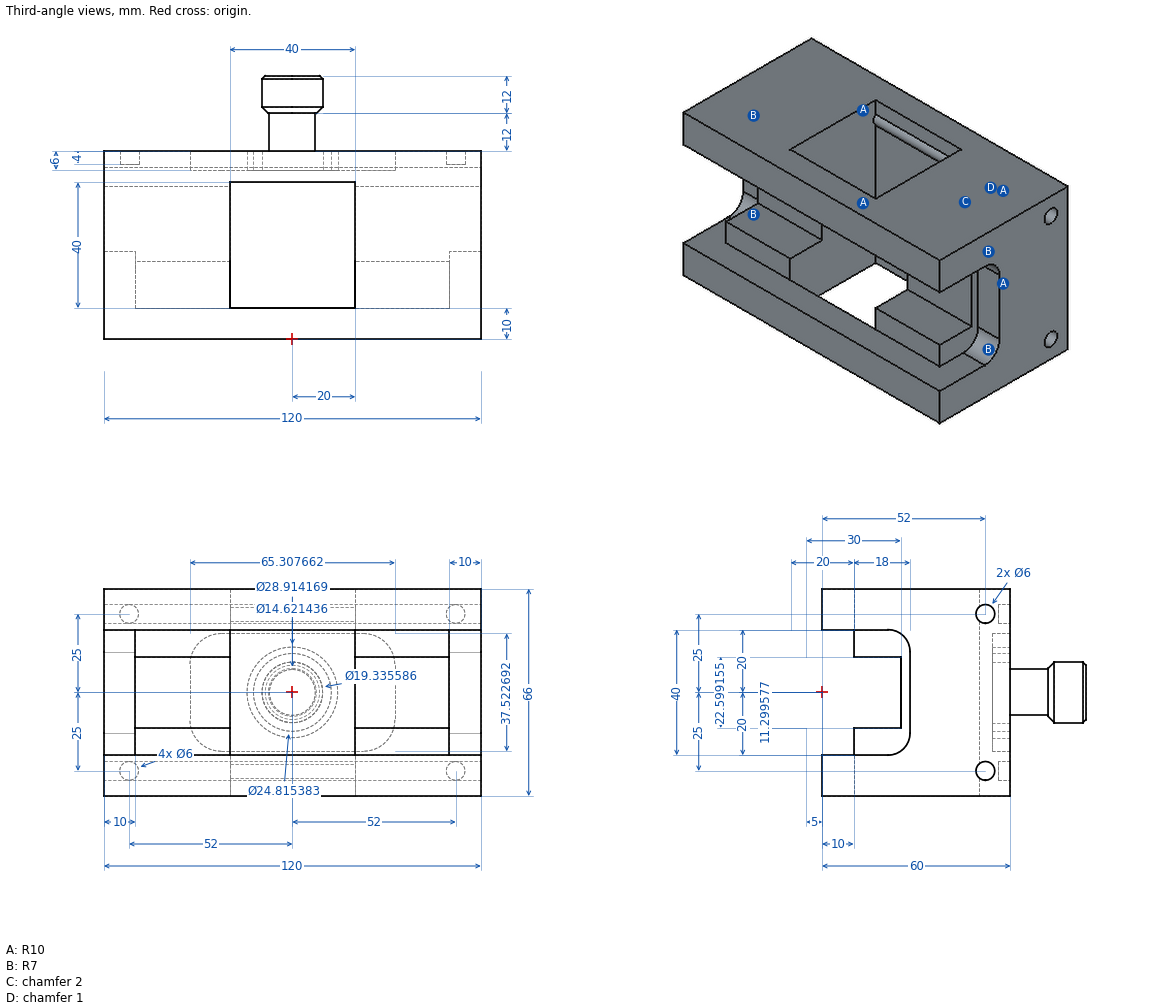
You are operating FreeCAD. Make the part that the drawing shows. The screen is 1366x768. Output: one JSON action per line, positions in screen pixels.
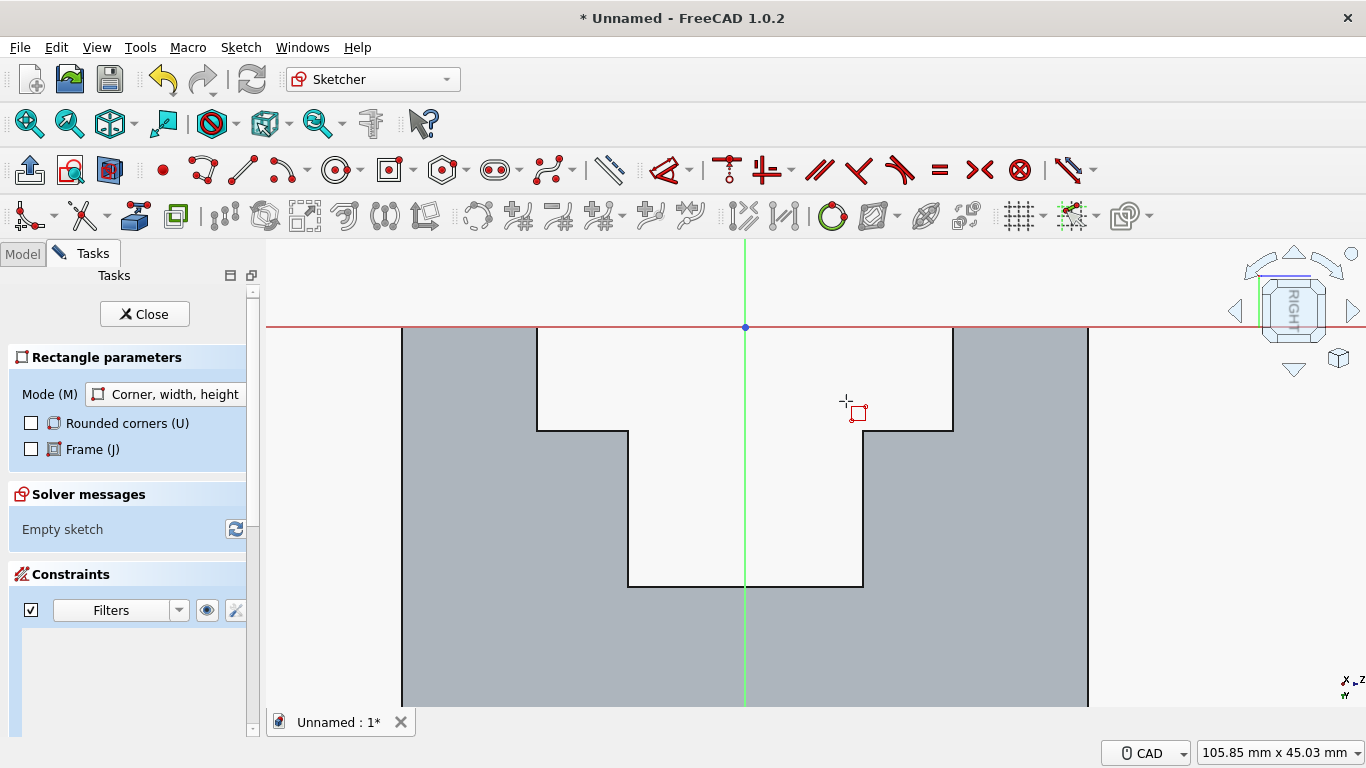
{"action": "left_click", "coordinate": [537, 431]}
{"action": "mouse_move", "coordinate": [953, 618]}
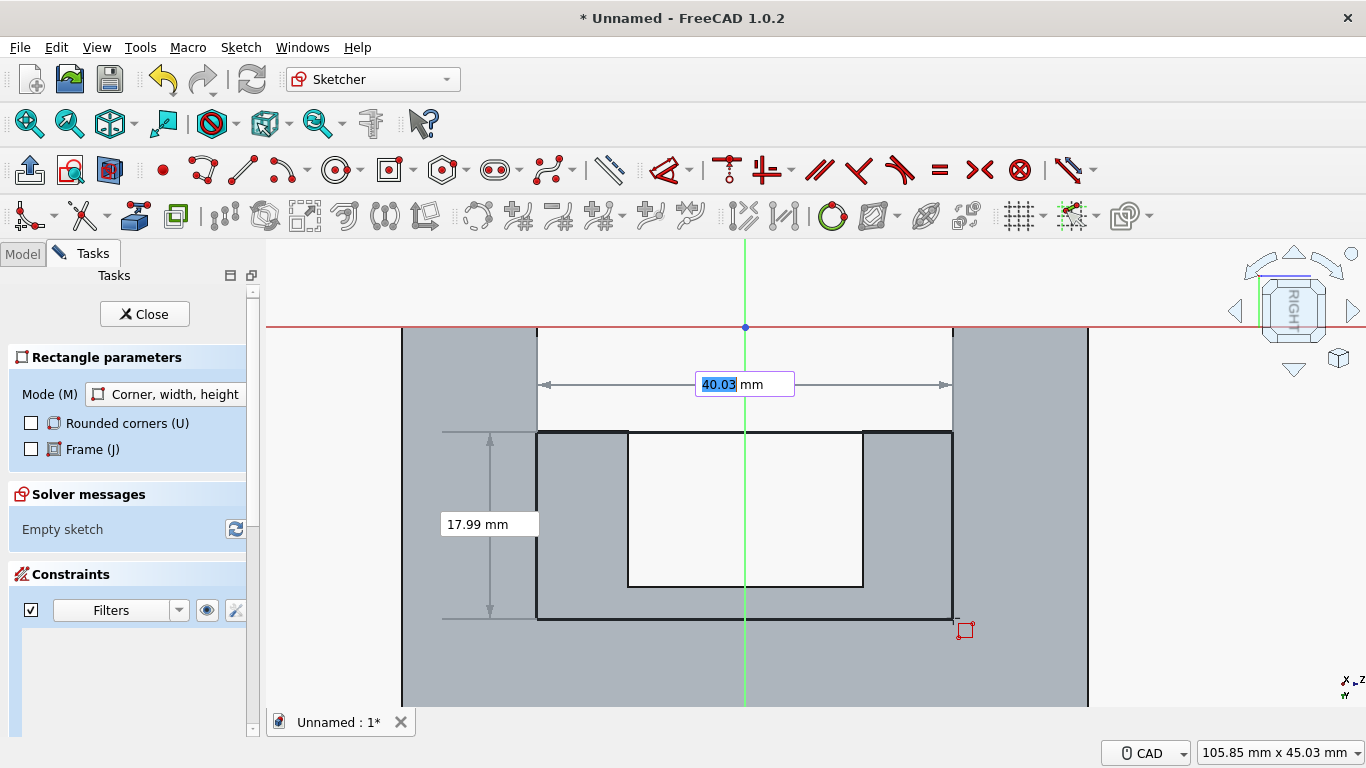
{"action": "type", "text": "40"}
{"action": "key", "text": "Tab"}
{"action": "type", "text": "18"}
{"action": "key", "text": "Return"}
{"action": "key", "text": "Escape"}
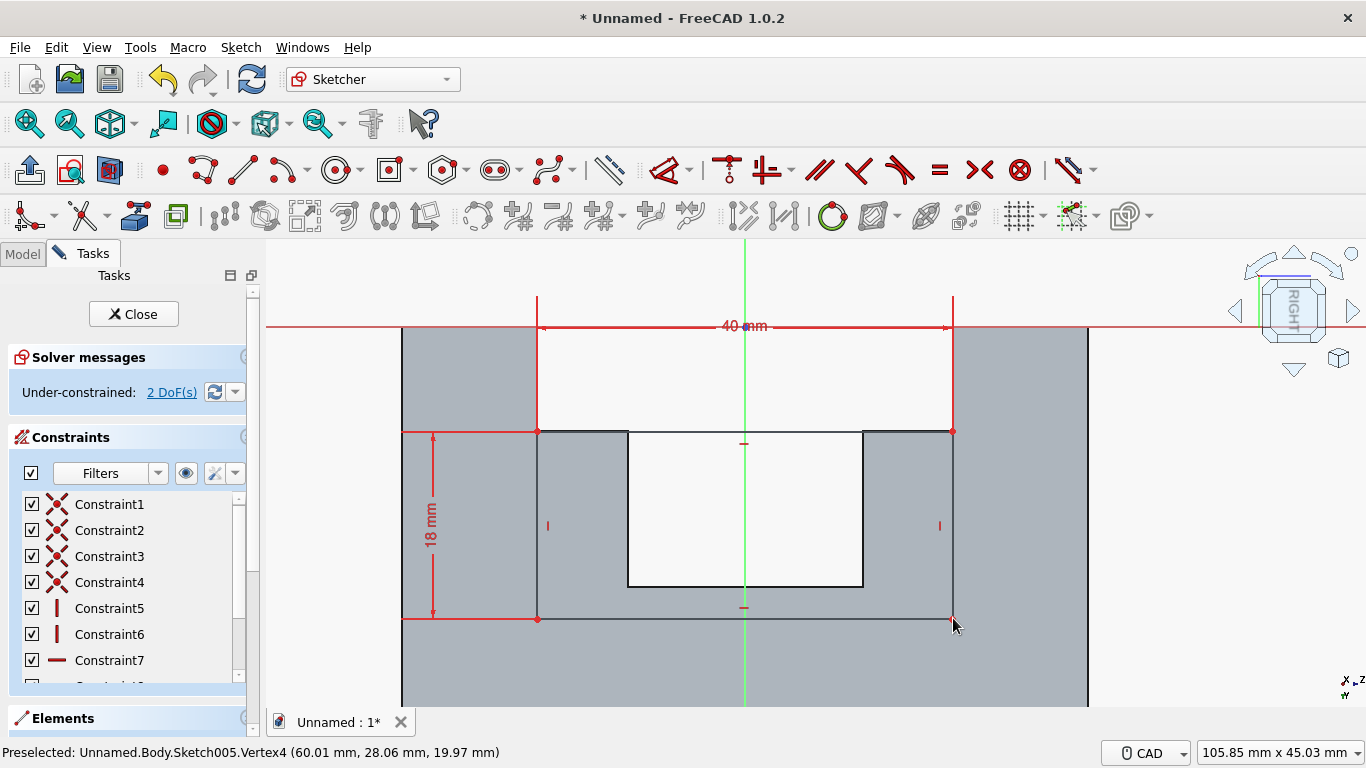
{"action": "left_click", "coordinate": [664, 170]}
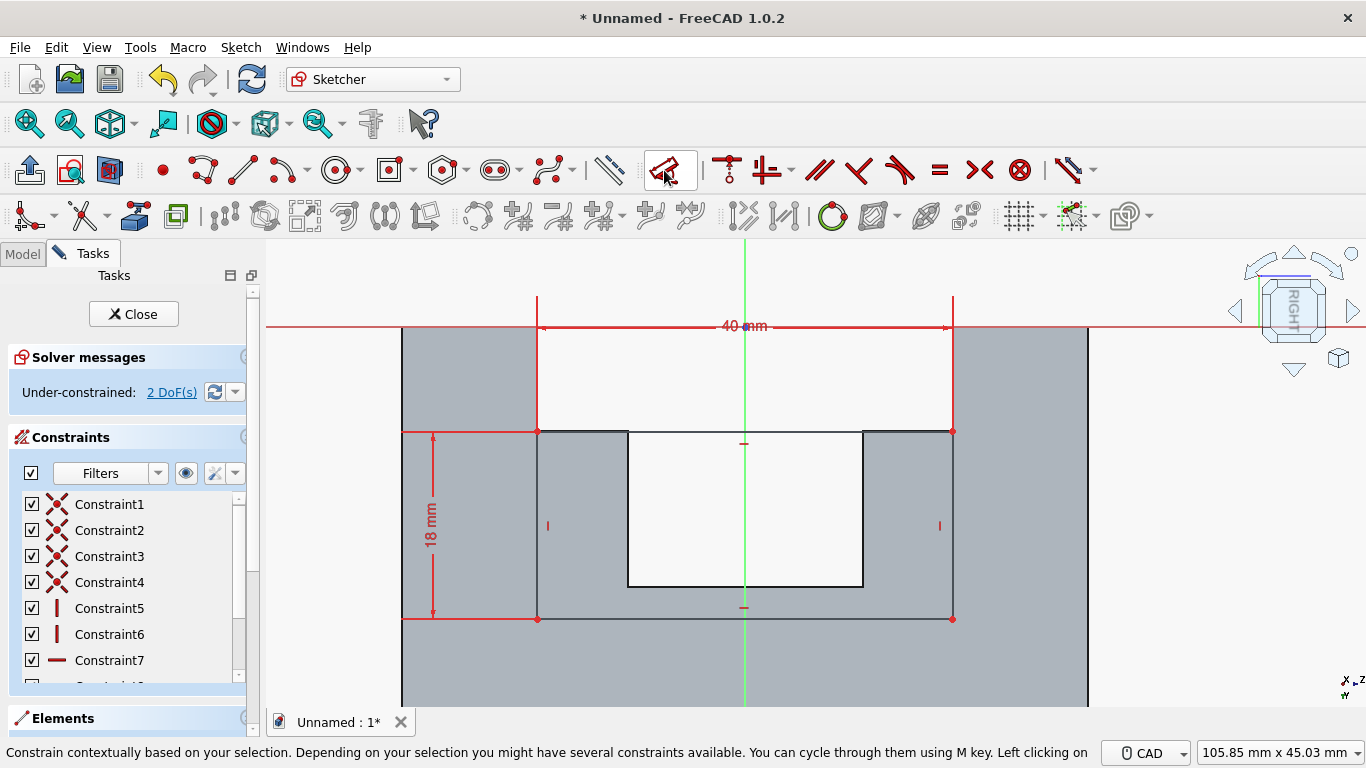
{"action": "left_click", "coordinate": [537, 432]}
{"action": "left_click", "coordinate": [641, 293]}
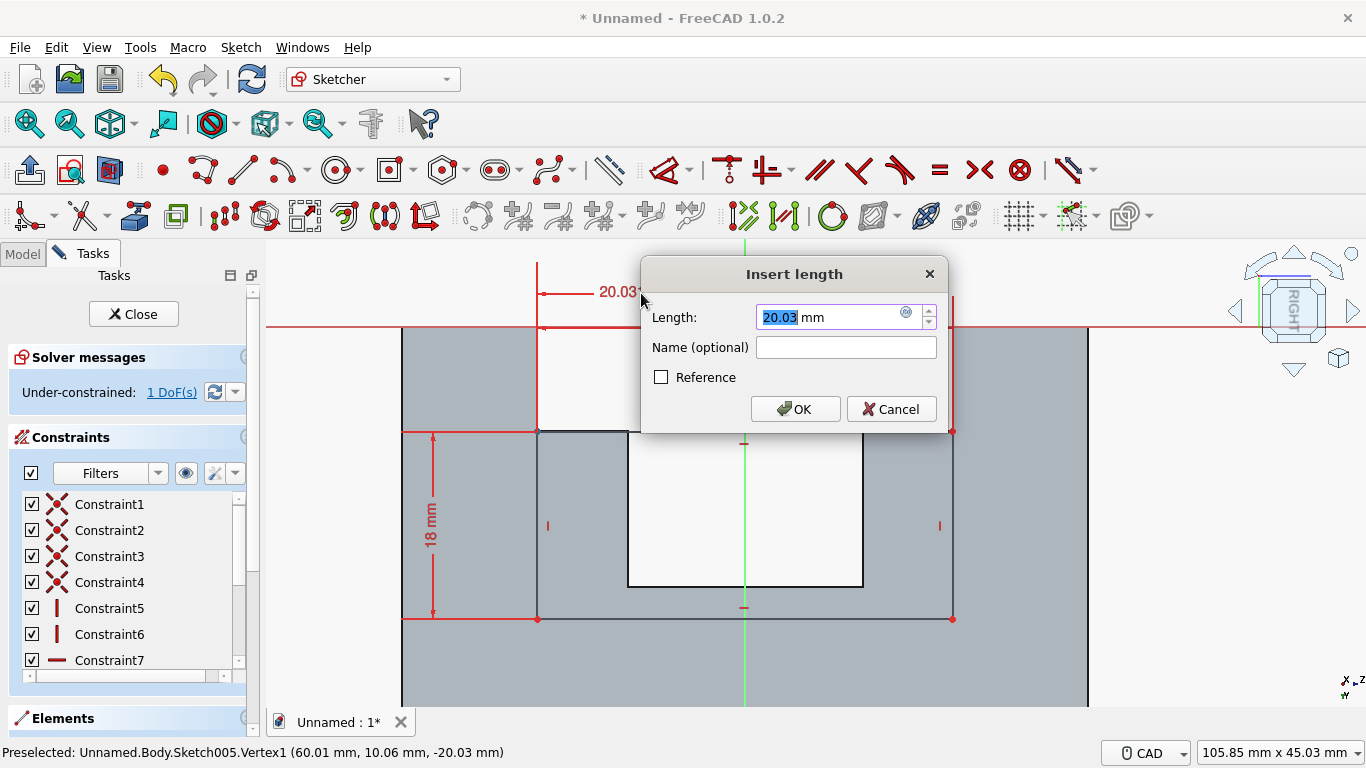
{"action": "type", "text": "20"}
{"action": "key", "text": "Return"}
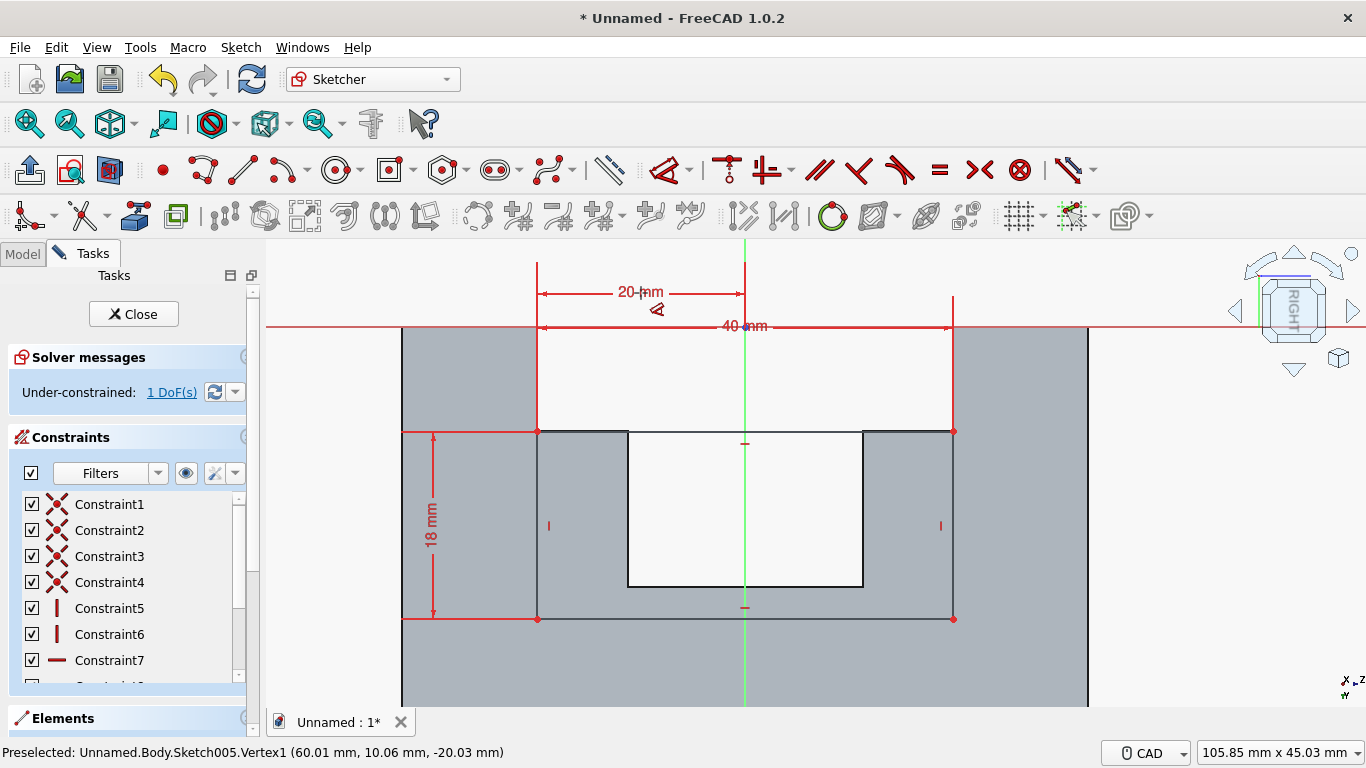
{"action": "left_click", "coordinate": [537, 432]}
{"action": "left_click", "coordinate": [503, 380]}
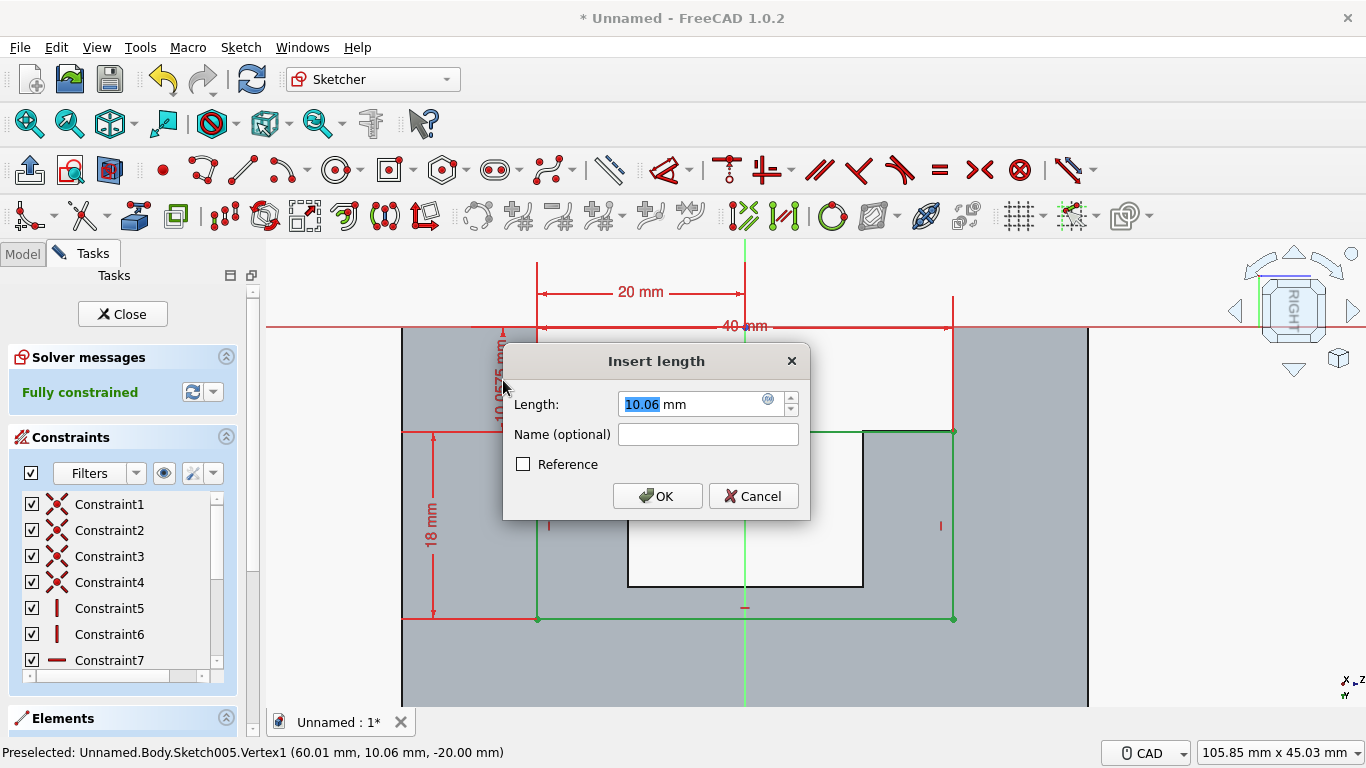
{"action": "type", "text": "10"}
{"action": "key", "text": "Return"}
{"action": "key", "text": "Escape"}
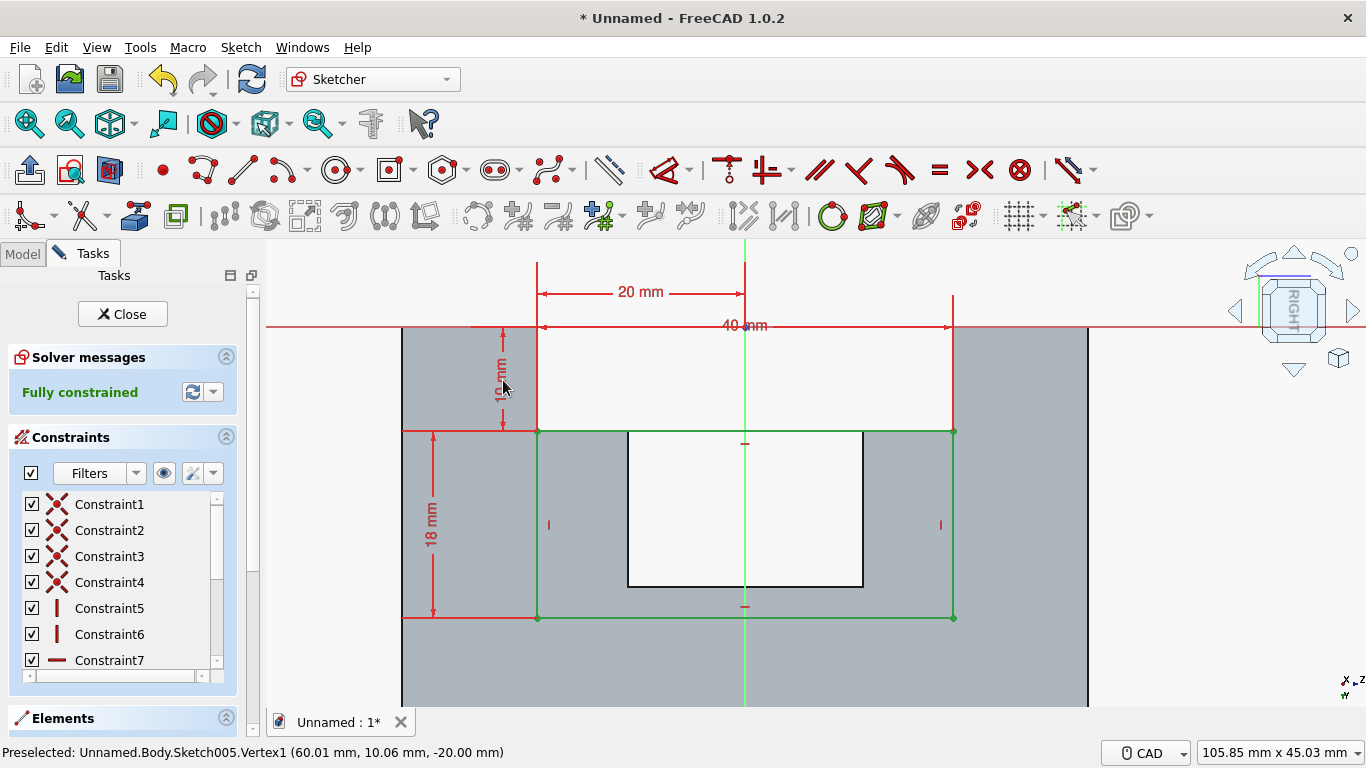
{"action": "left_click", "coordinate": [123, 314]}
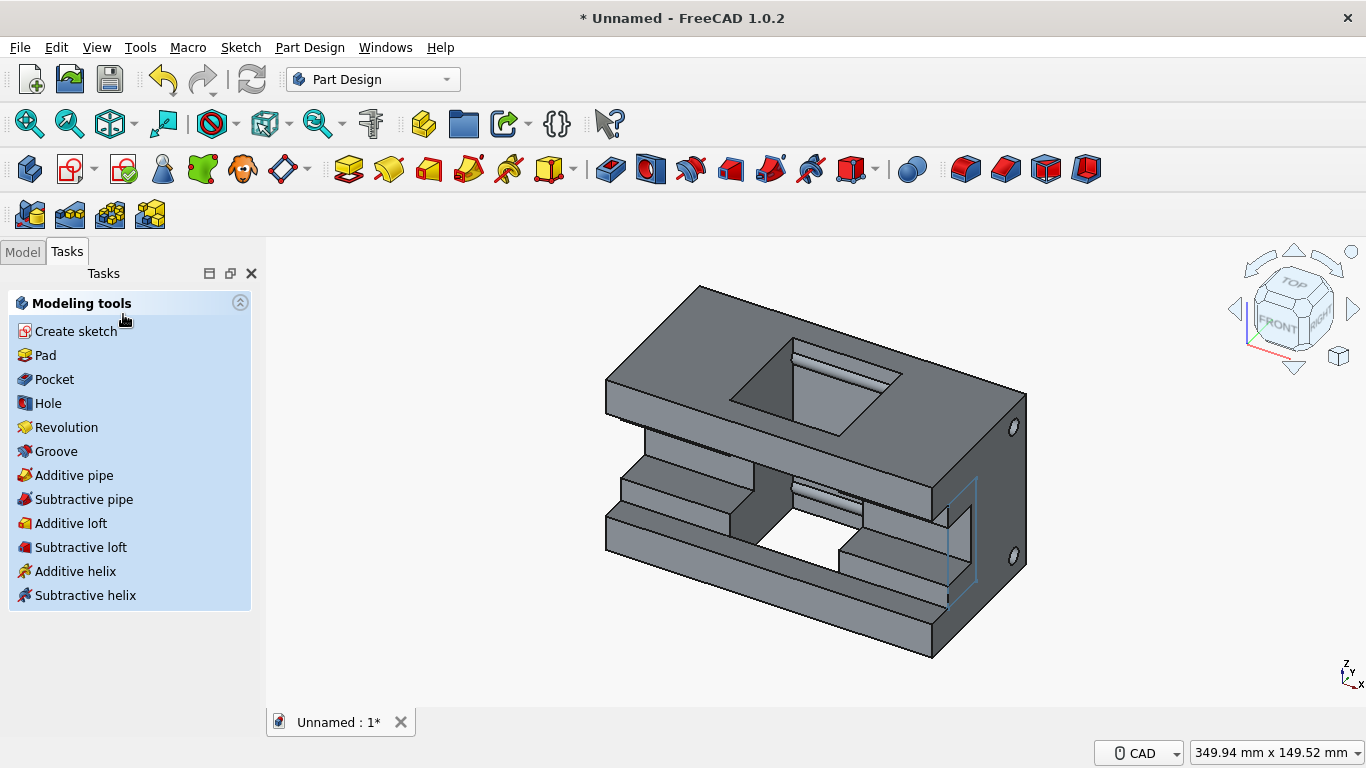
{"action": "left_click", "coordinate": [612, 170]}